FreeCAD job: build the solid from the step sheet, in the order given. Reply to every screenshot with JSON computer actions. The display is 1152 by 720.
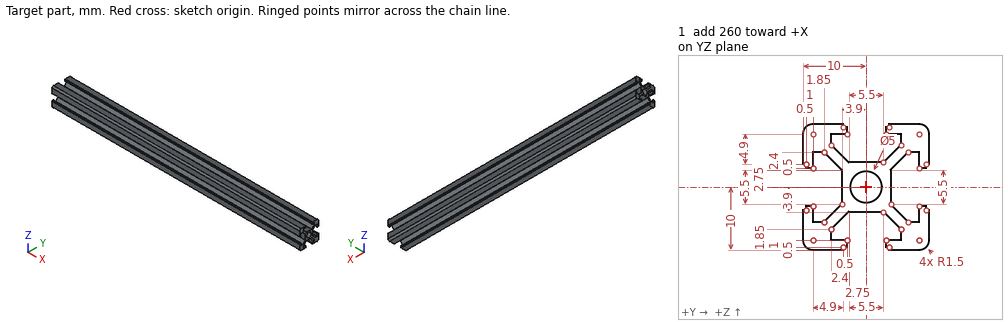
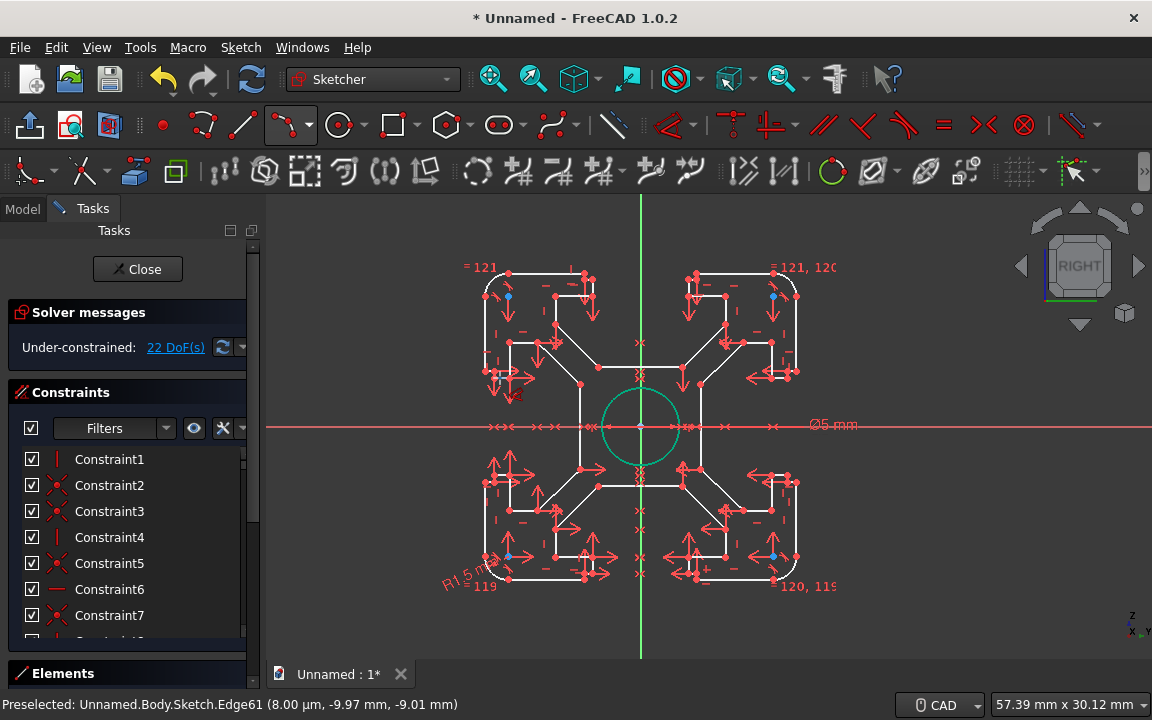
{"action": "left_click", "coordinate": [501, 378]}
{"action": "left_click", "coordinate": [505, 344]}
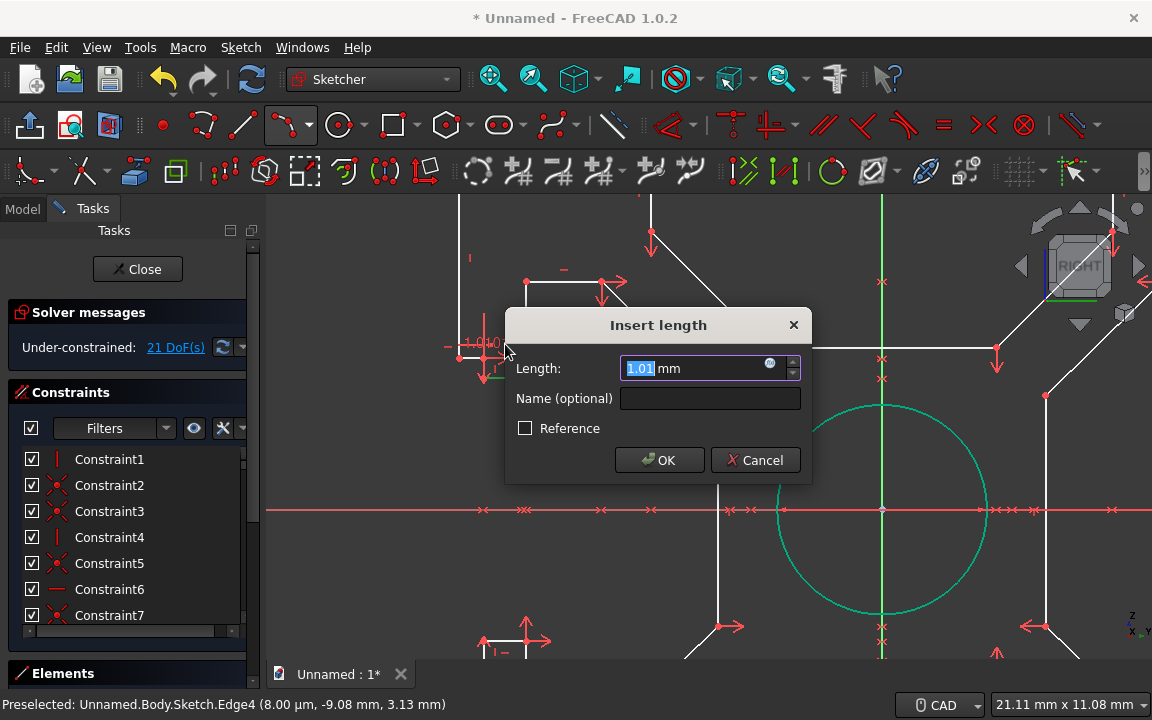
{"action": "type", "text": "1"}
{"action": "key", "text": "Return"}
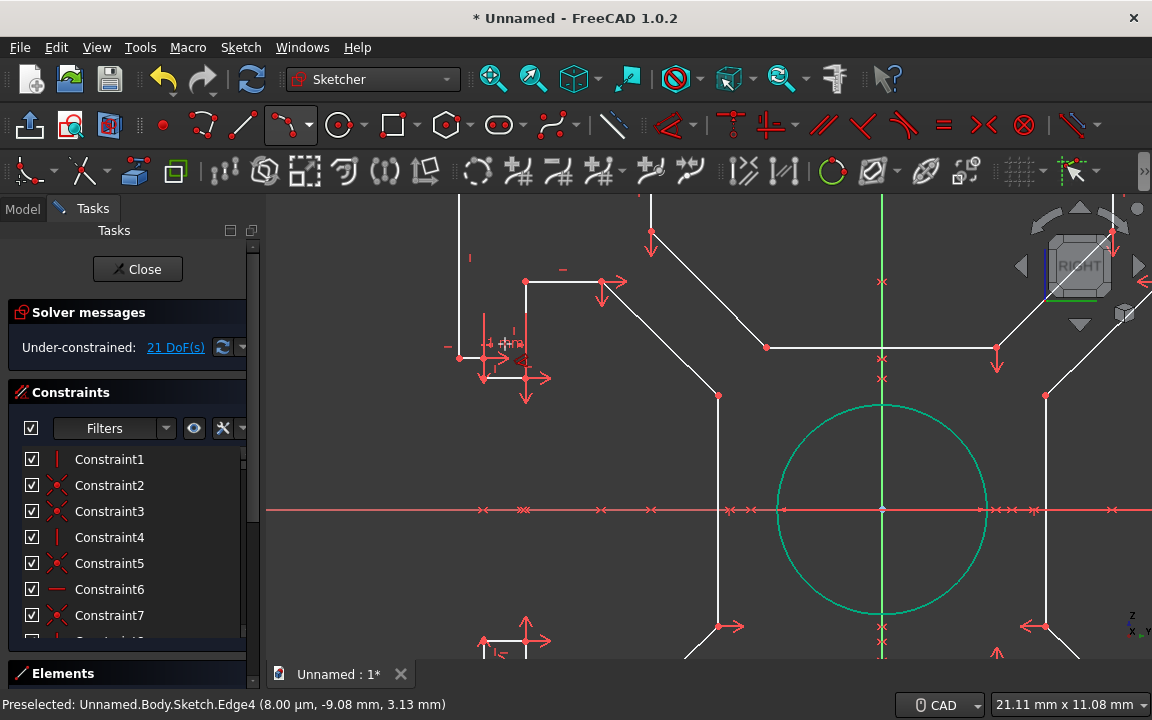
{"action": "scroll", "coordinate": [500, 378], "scroll_direction": "down", "scroll_amount": 5}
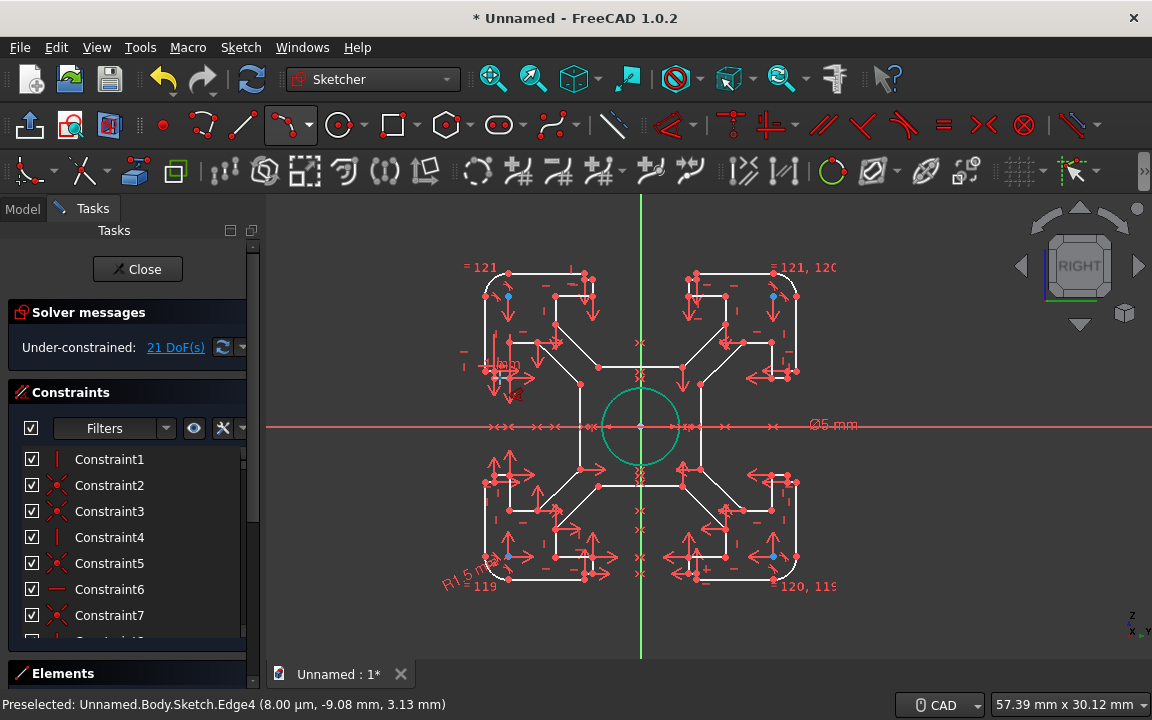
{"action": "scroll", "coordinate": [593, 569], "scroll_direction": "up", "scroll_amount": 6}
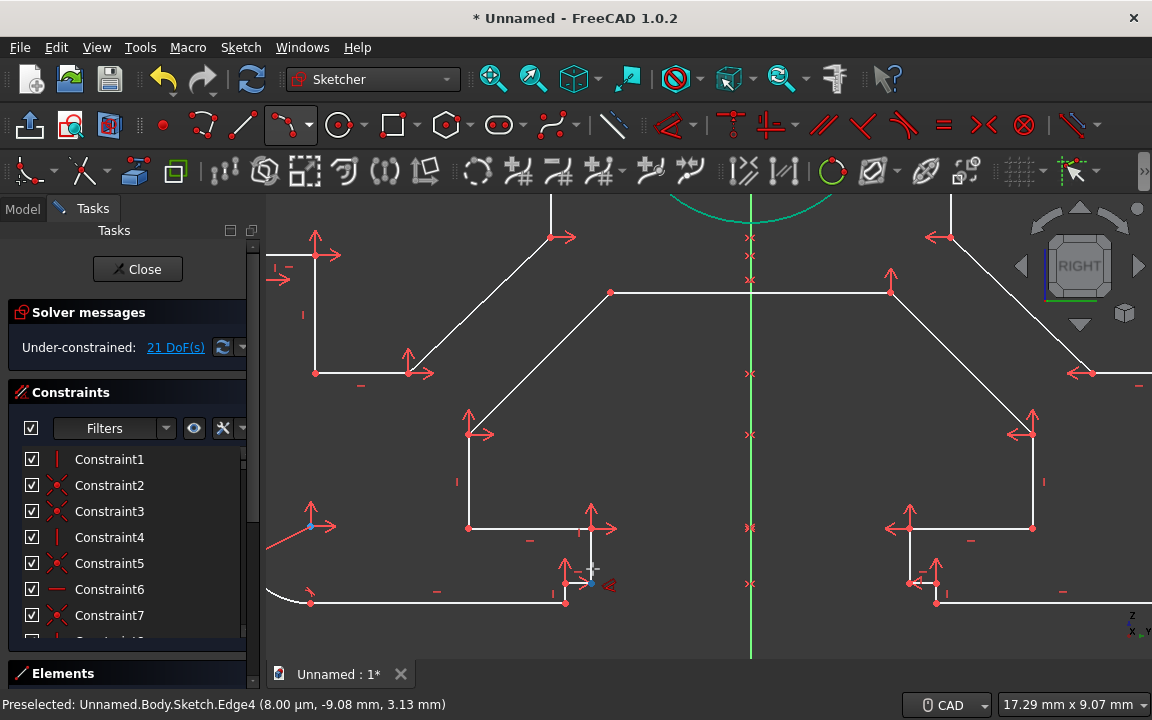
{"action": "left_click", "coordinate": [591, 567]}
{"action": "left_click", "coordinate": [557, 556]}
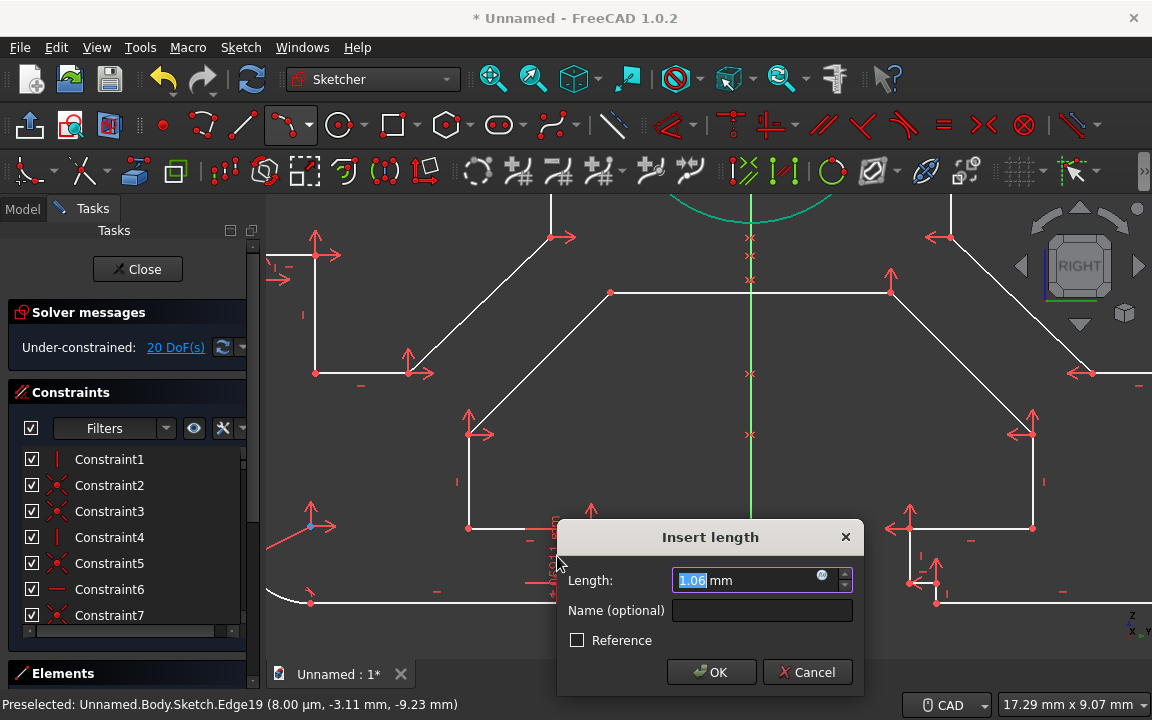
{"action": "type", "text": "1"}
{"action": "key", "text": "Return"}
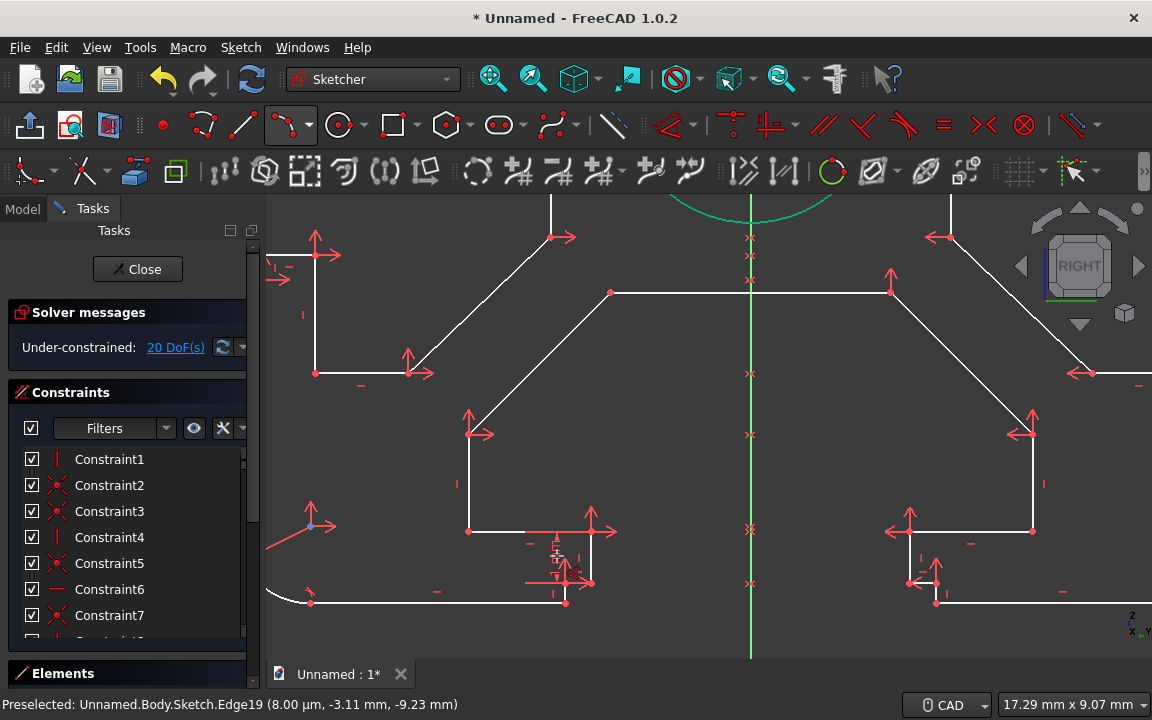
{"action": "scroll", "coordinate": [593, 569], "scroll_direction": "down", "scroll_amount": 6}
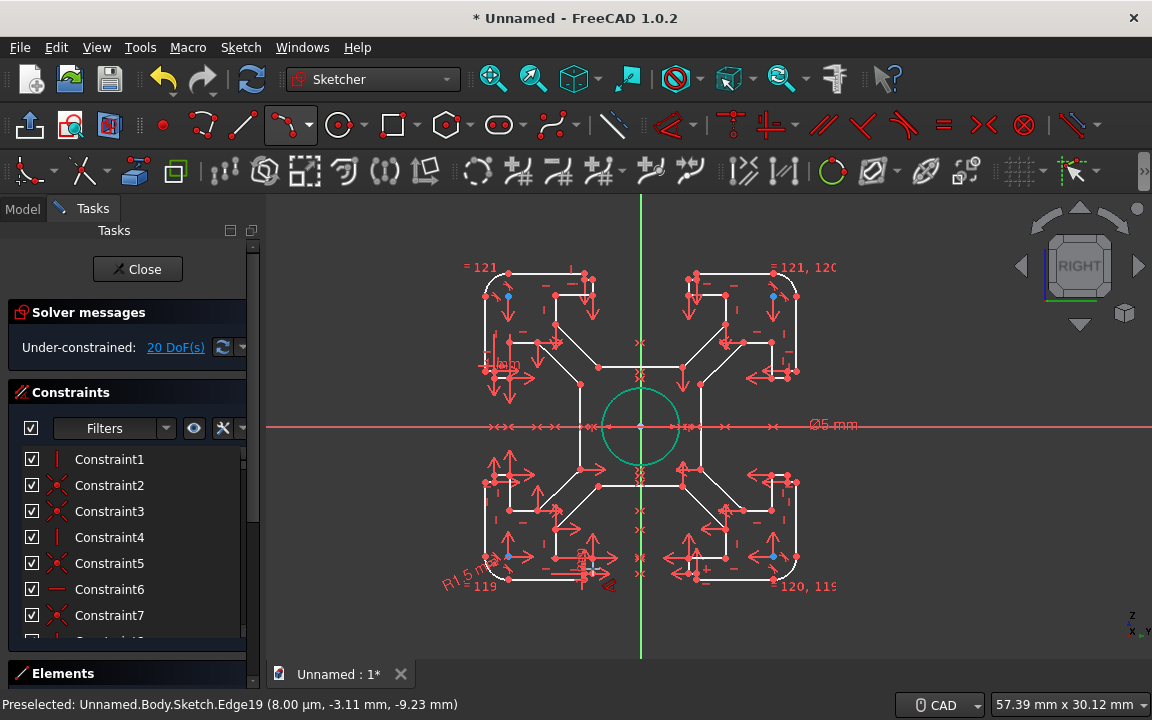
{"action": "left_click", "coordinate": [485, 319]}
{"action": "left_click", "coordinate": [451, 334]}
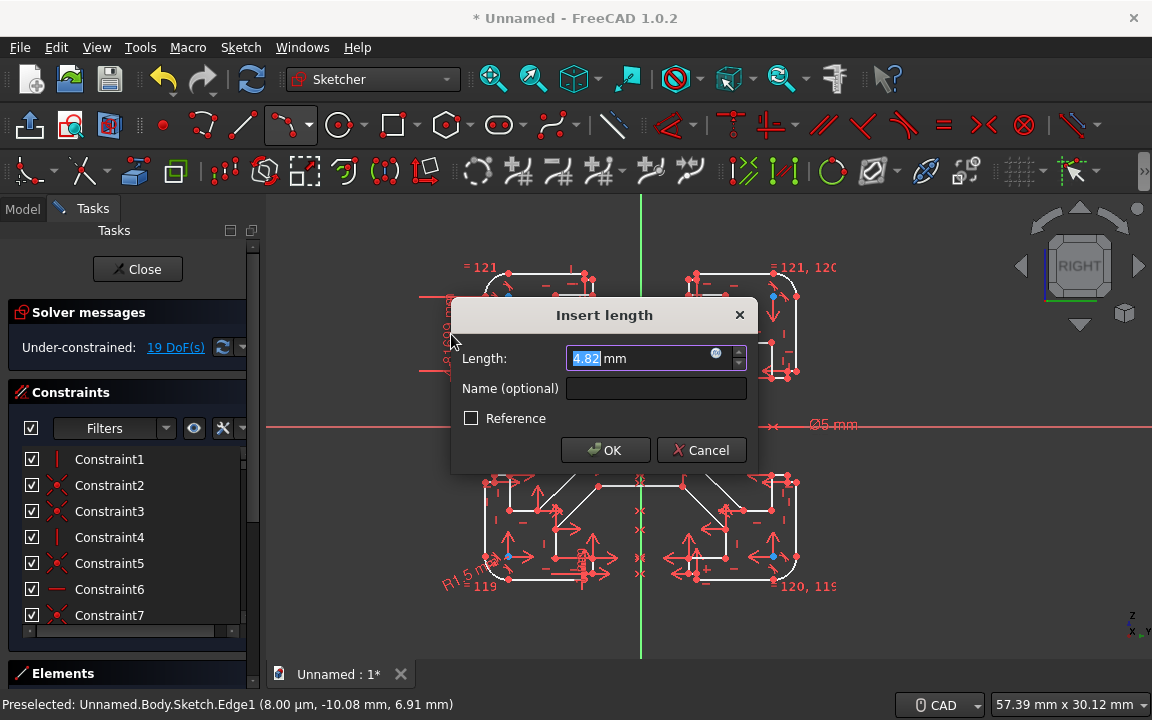
{"action": "type", "text": "4.9"}
{"action": "key", "text": "Return"}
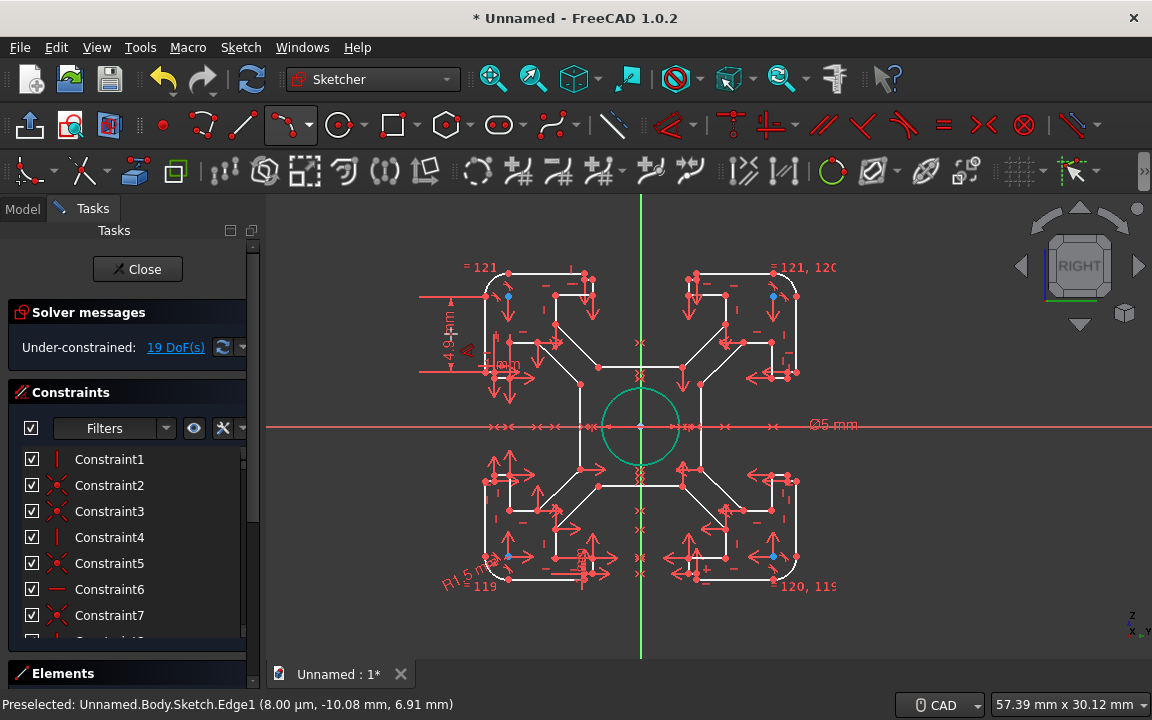
{"action": "scroll", "coordinate": [490, 372], "scroll_direction": "up", "scroll_amount": 9}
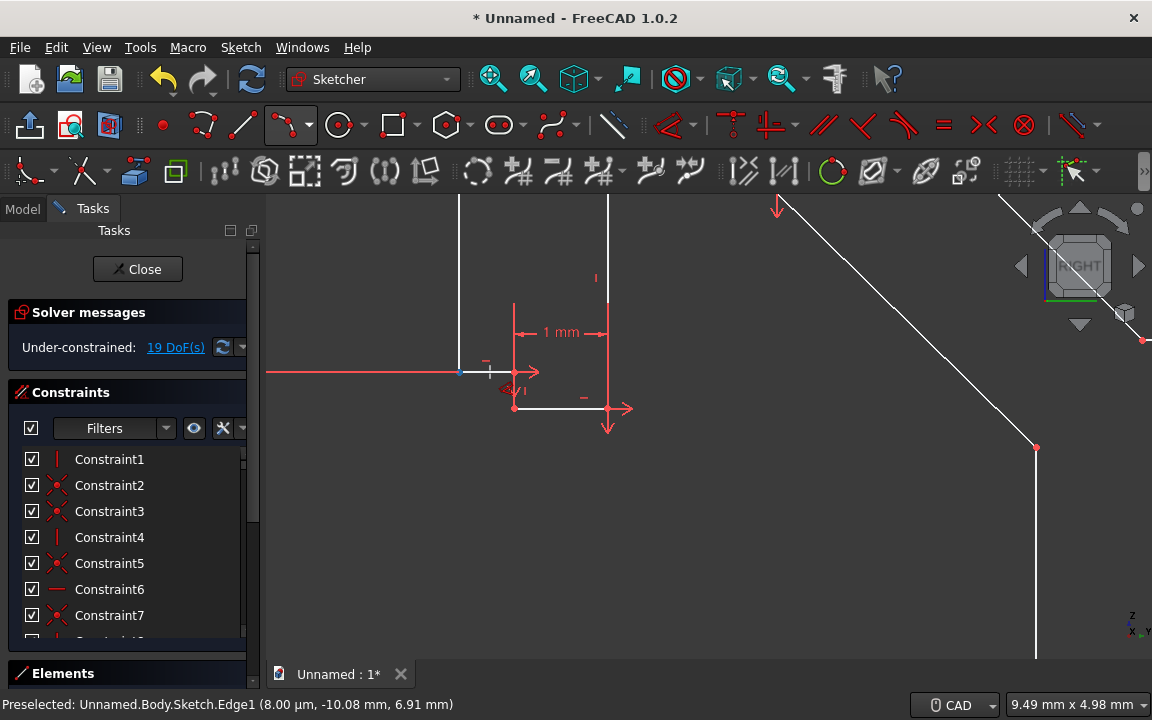
{"action": "left_click", "coordinate": [487, 372]}
{"action": "left_click", "coordinate": [487, 338]}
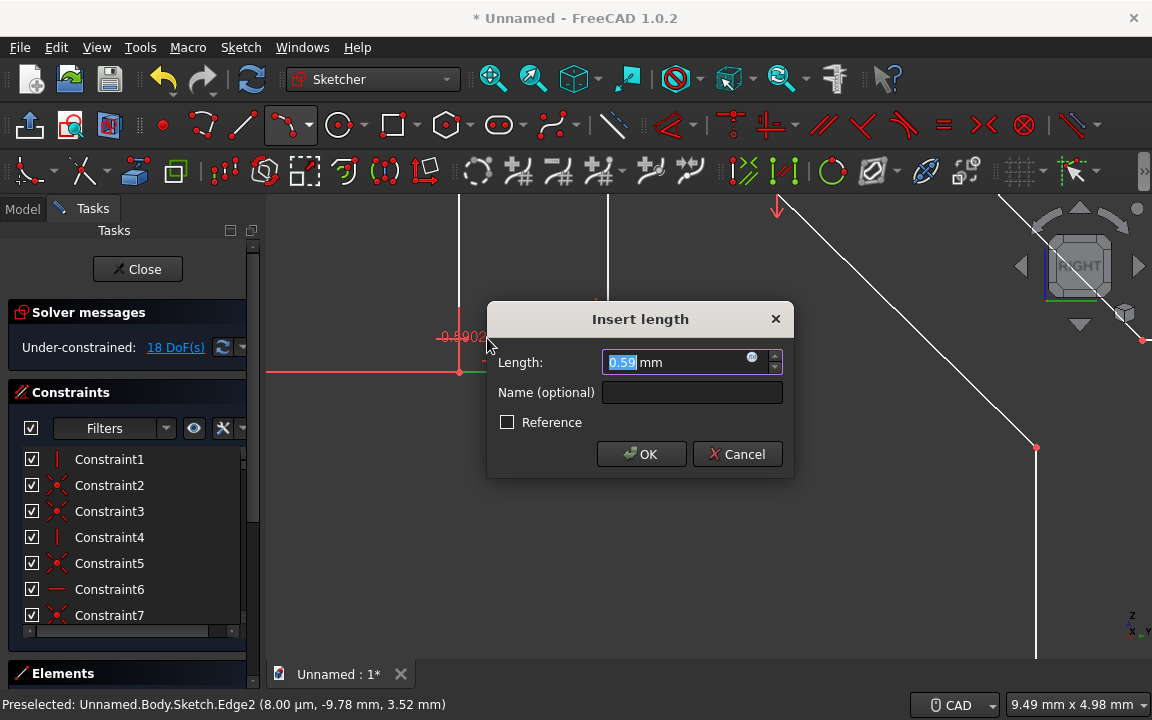
{"action": "type", "text": "0.5"}
{"action": "key", "text": "Return"}